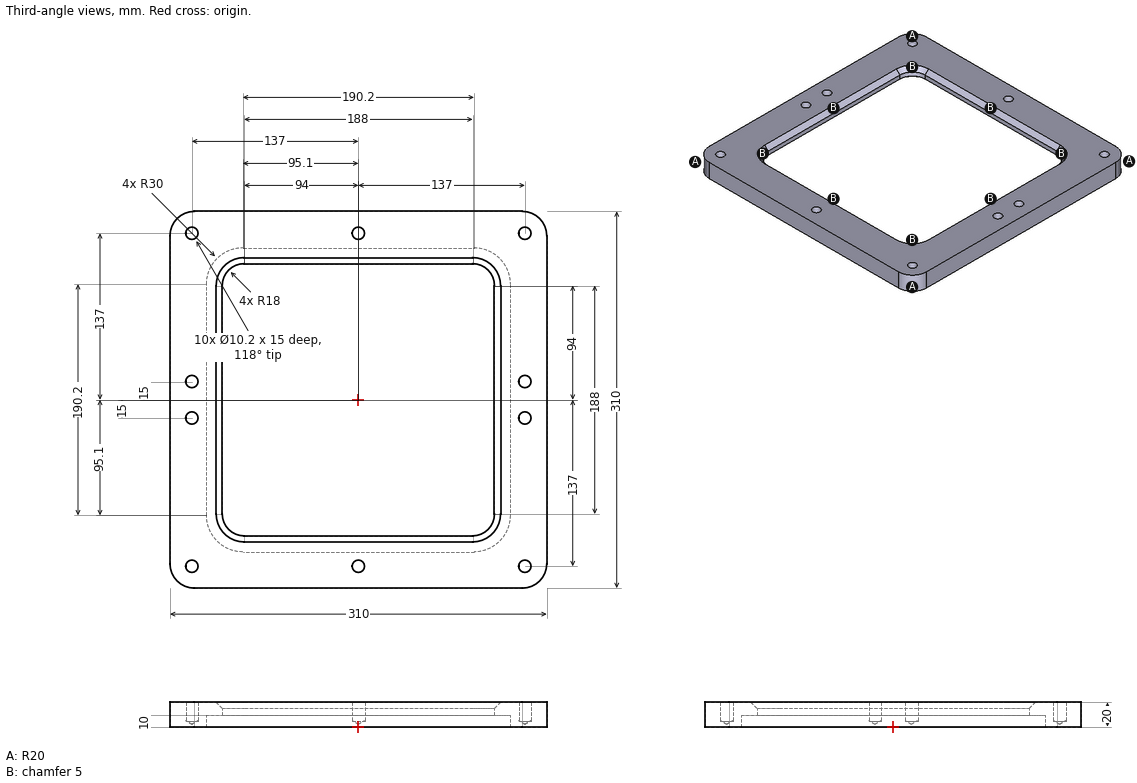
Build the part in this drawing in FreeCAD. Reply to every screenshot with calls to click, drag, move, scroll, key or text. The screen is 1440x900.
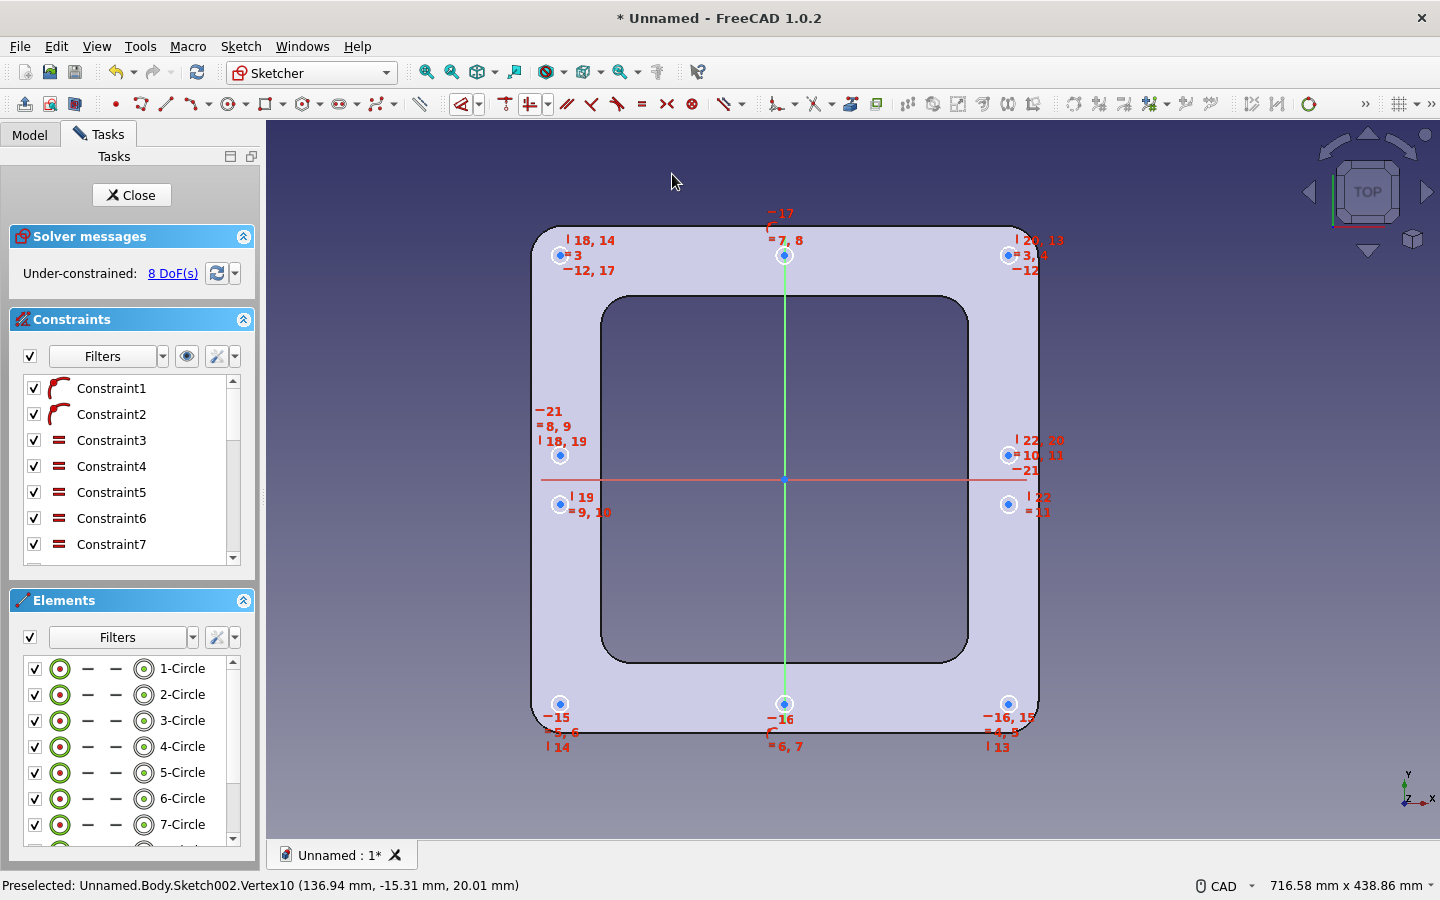
click(560, 505)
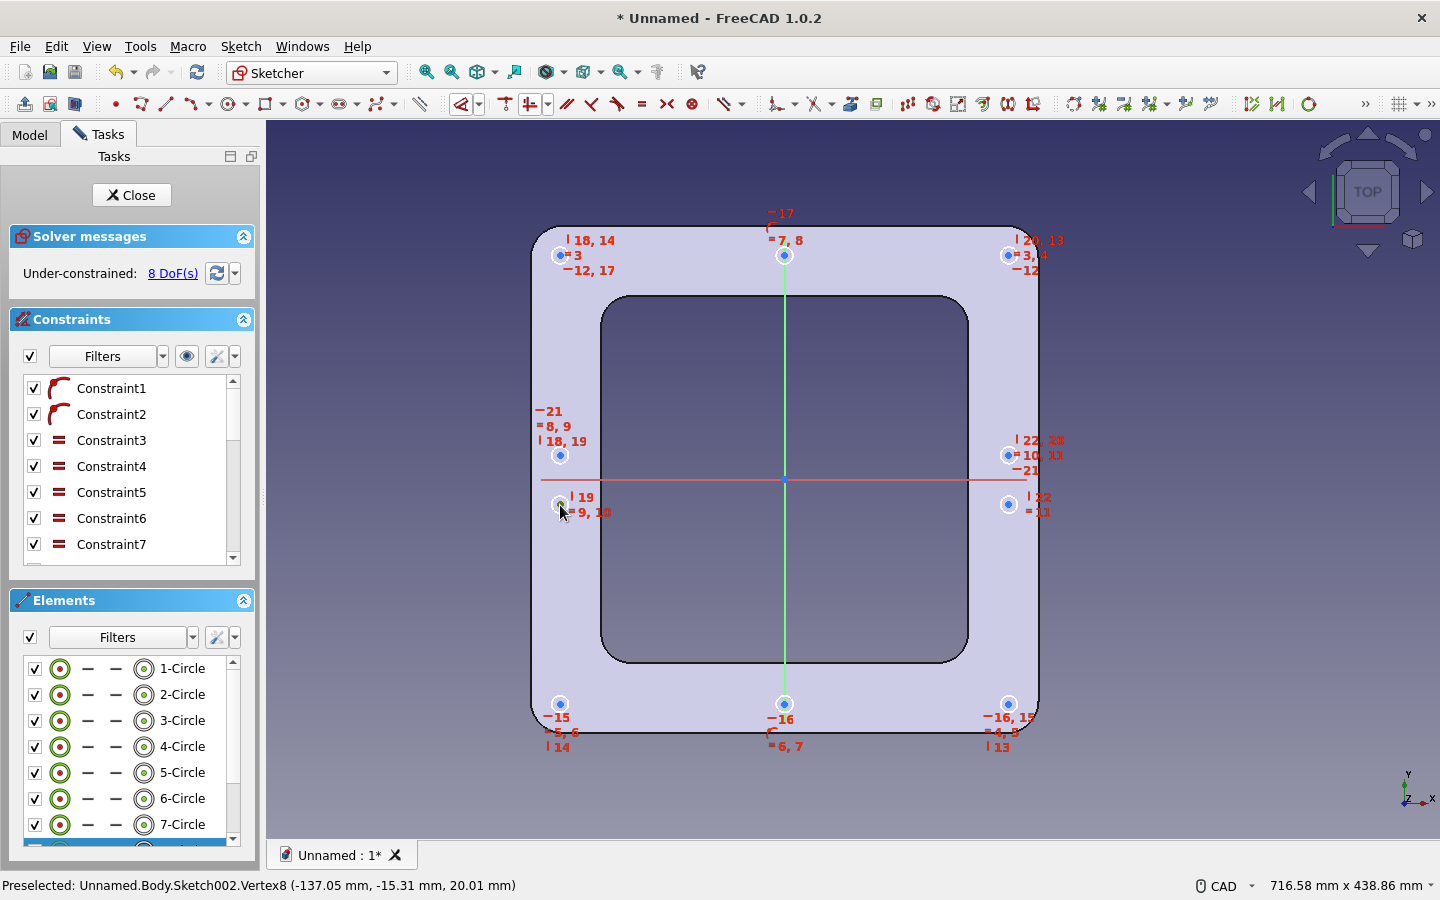
click(1009, 505)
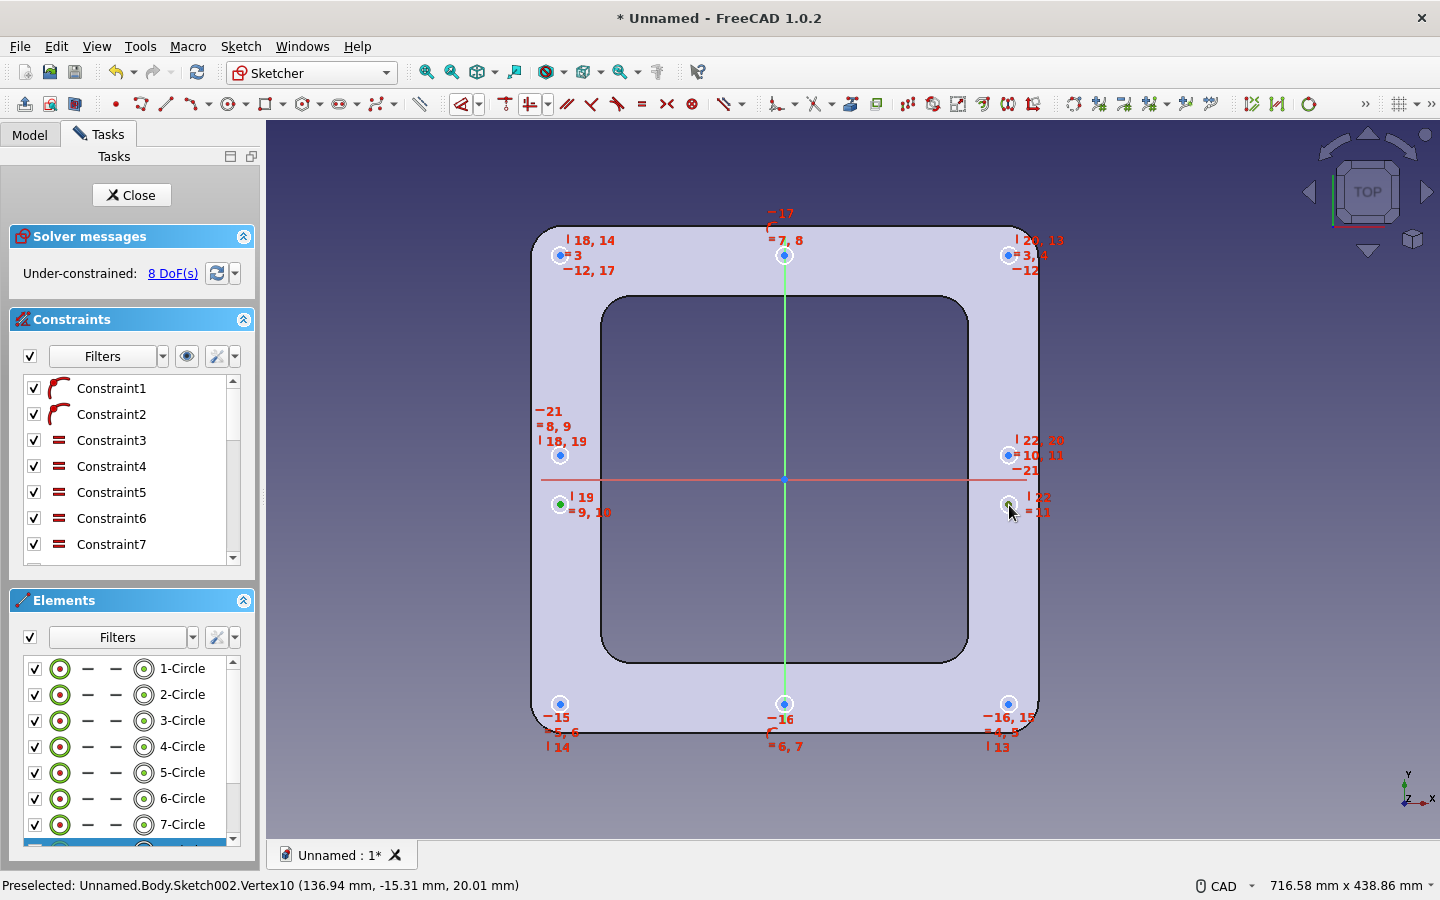
click(548, 104)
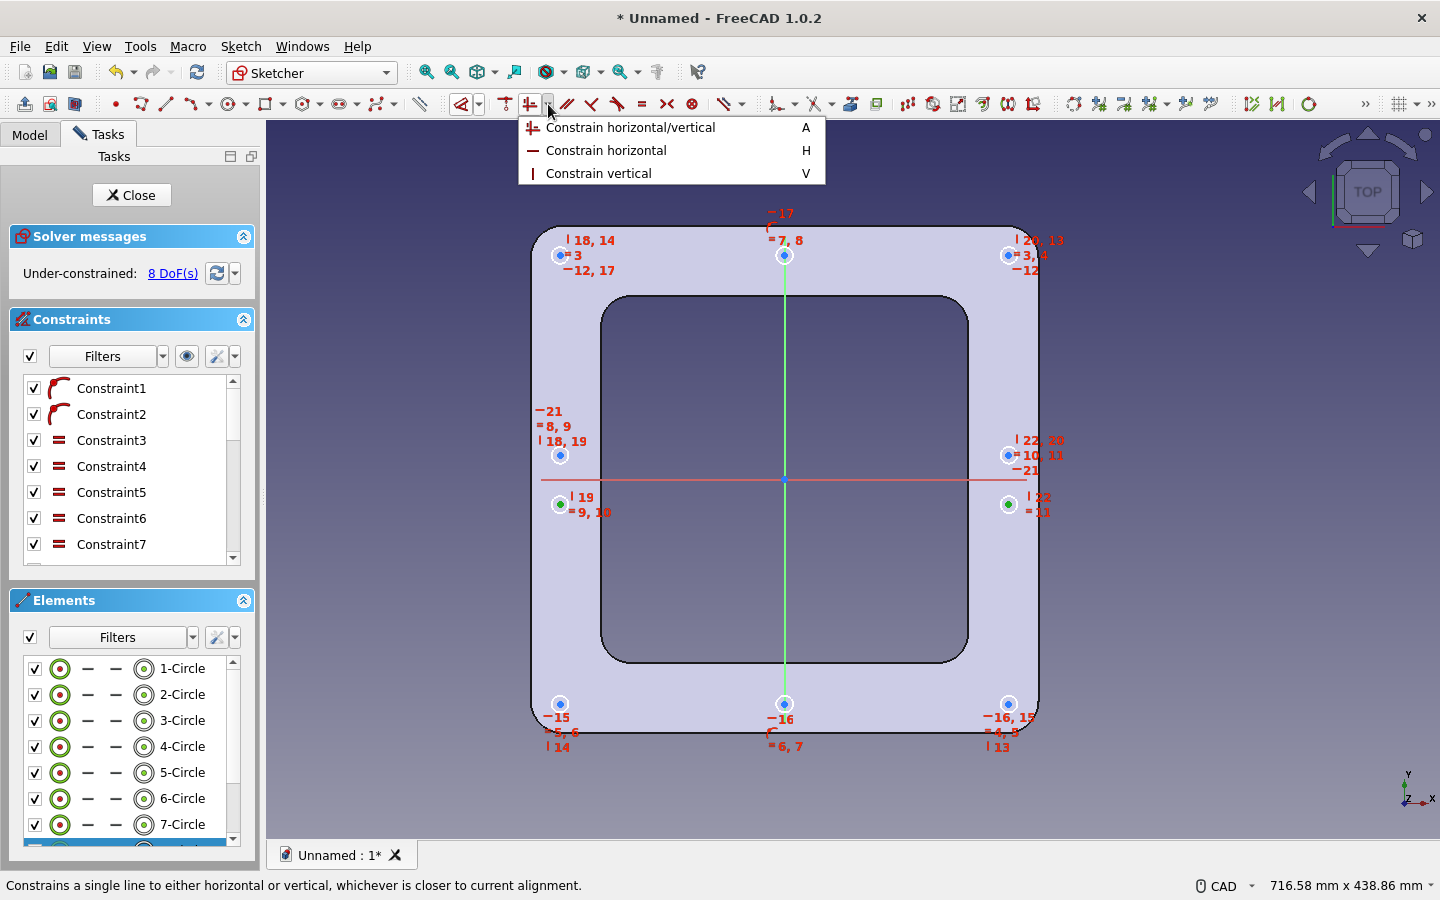
click(672, 150)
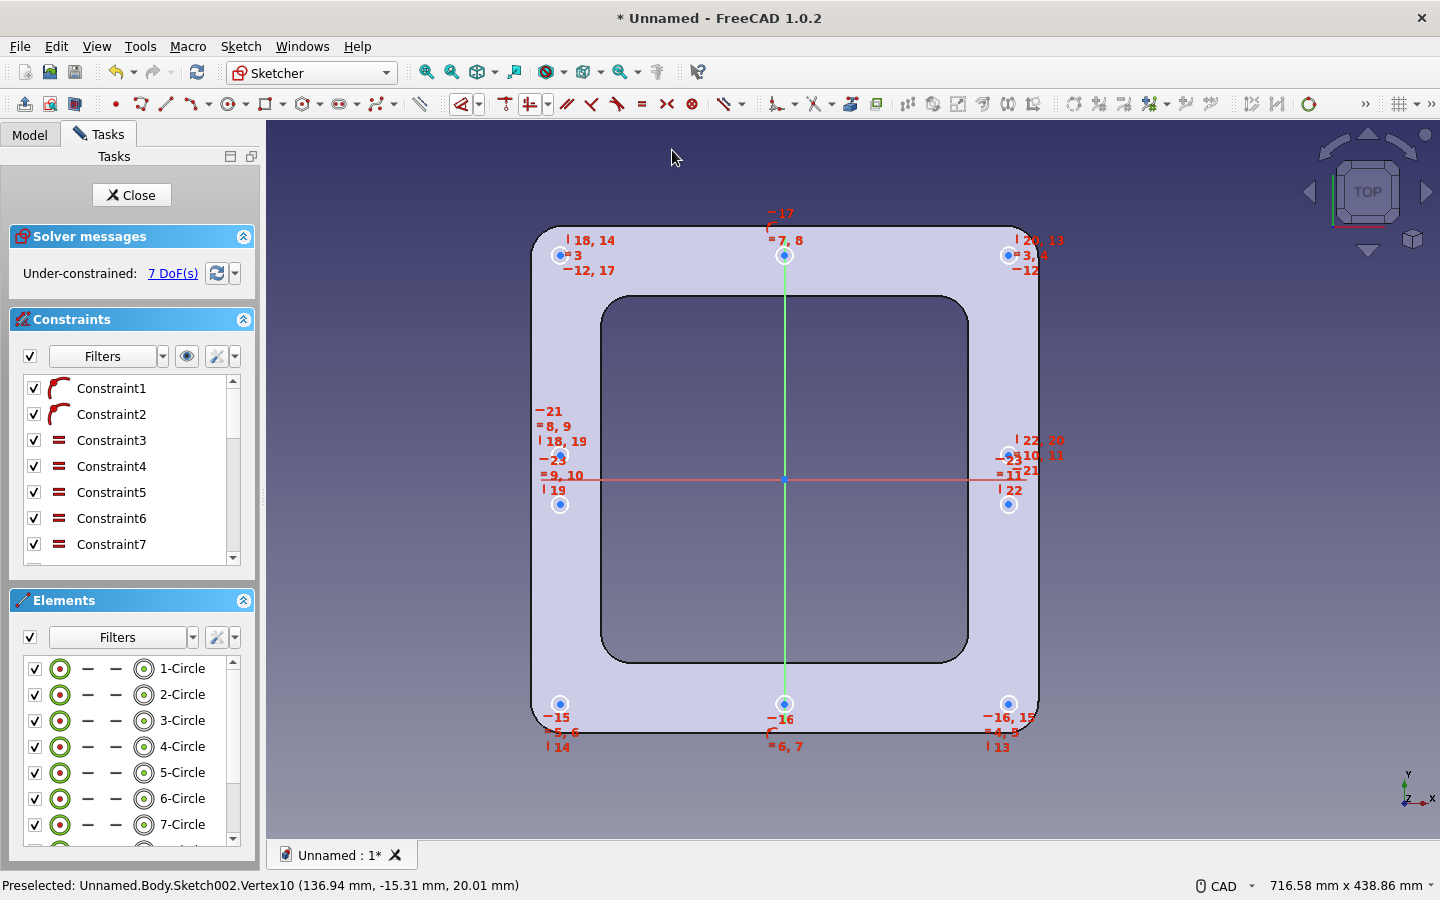
scroll(560, 247, up, 5)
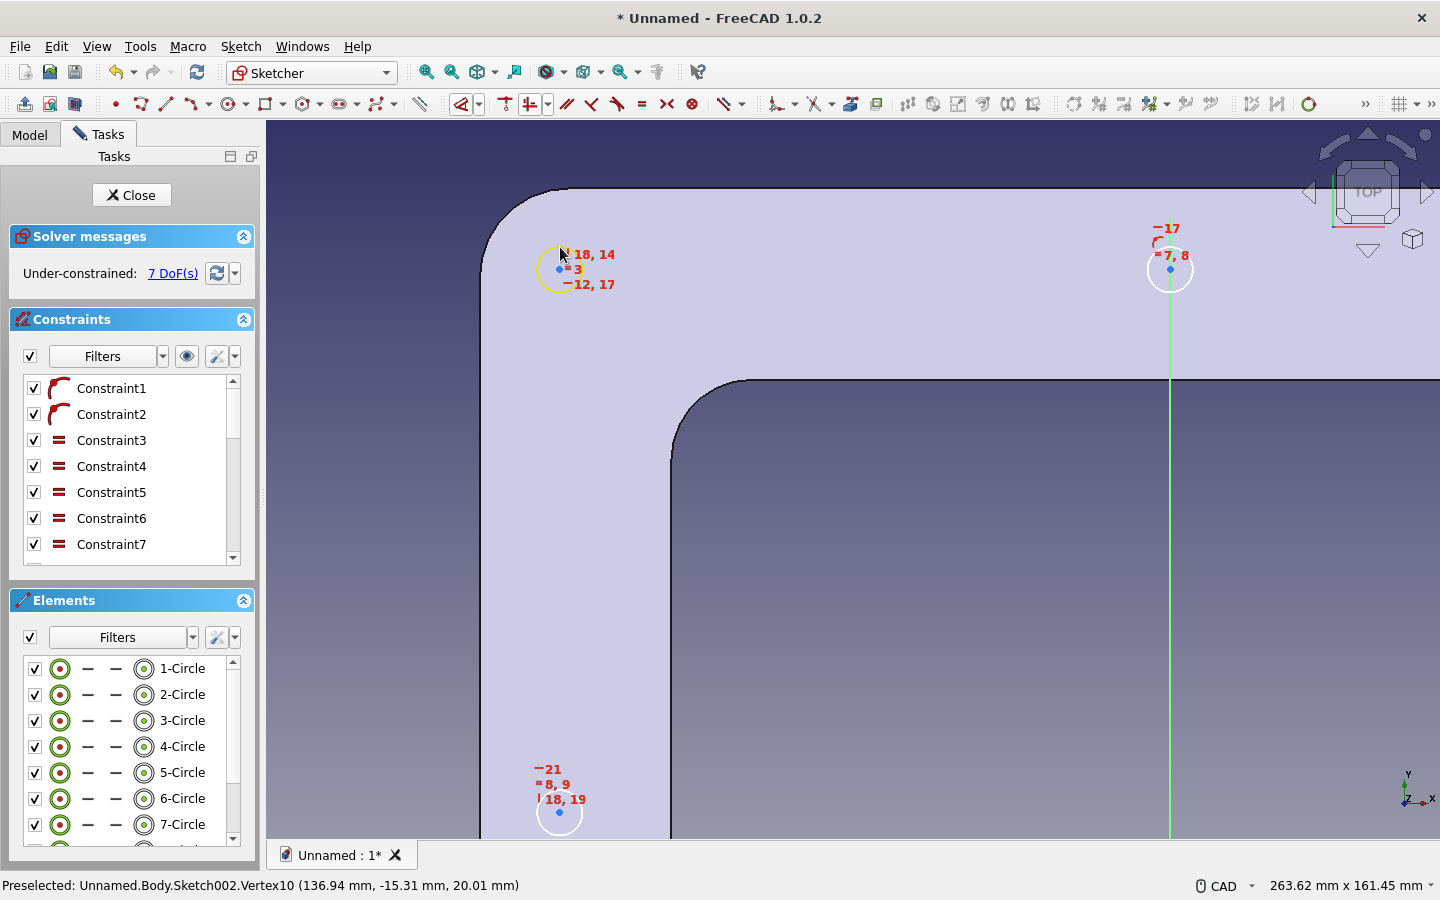
click(560, 247)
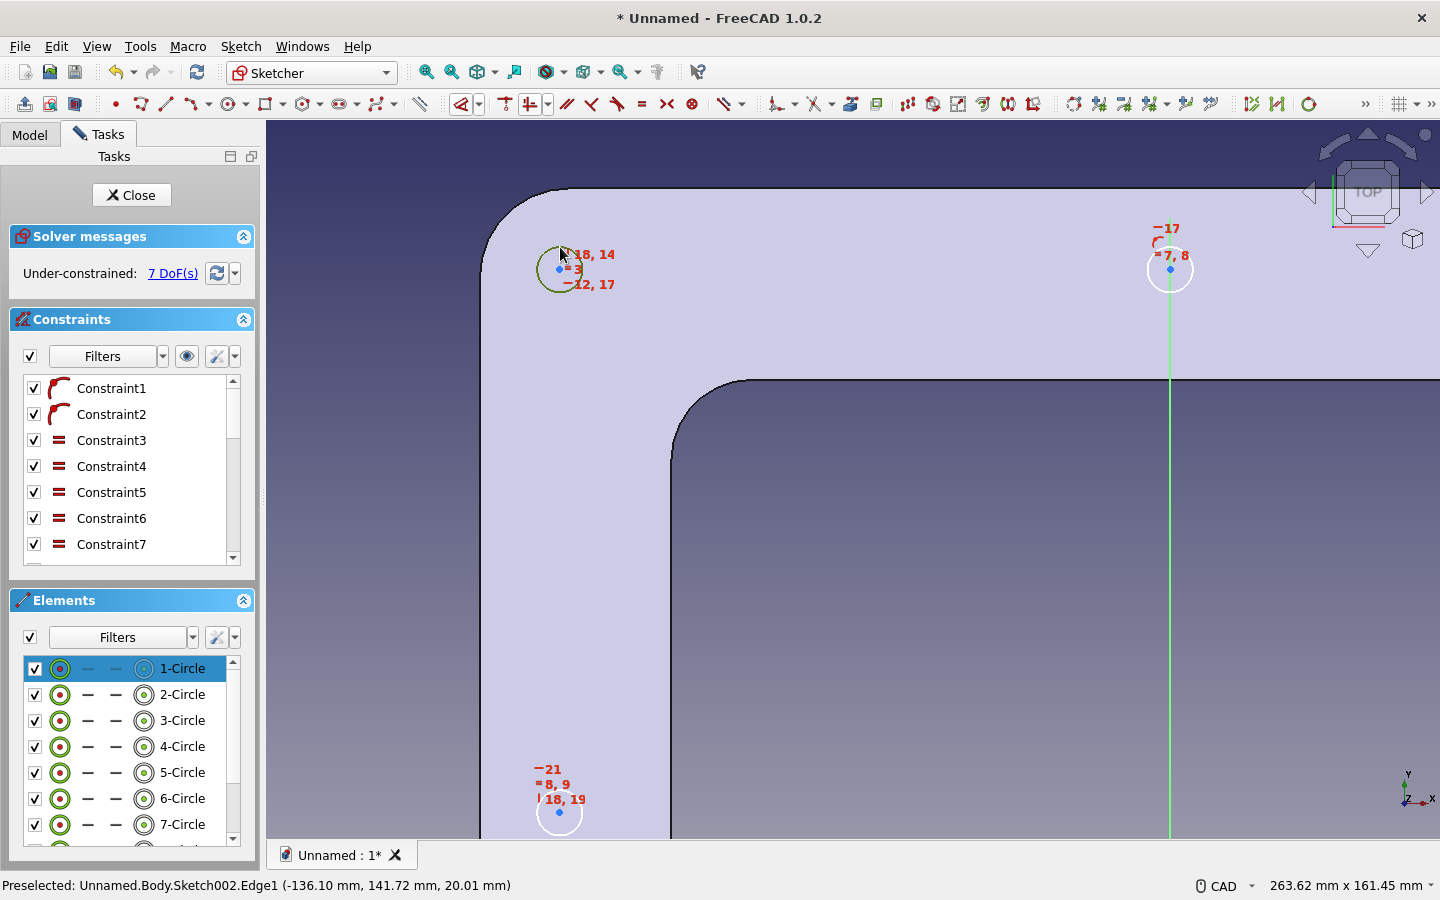
click(478, 104)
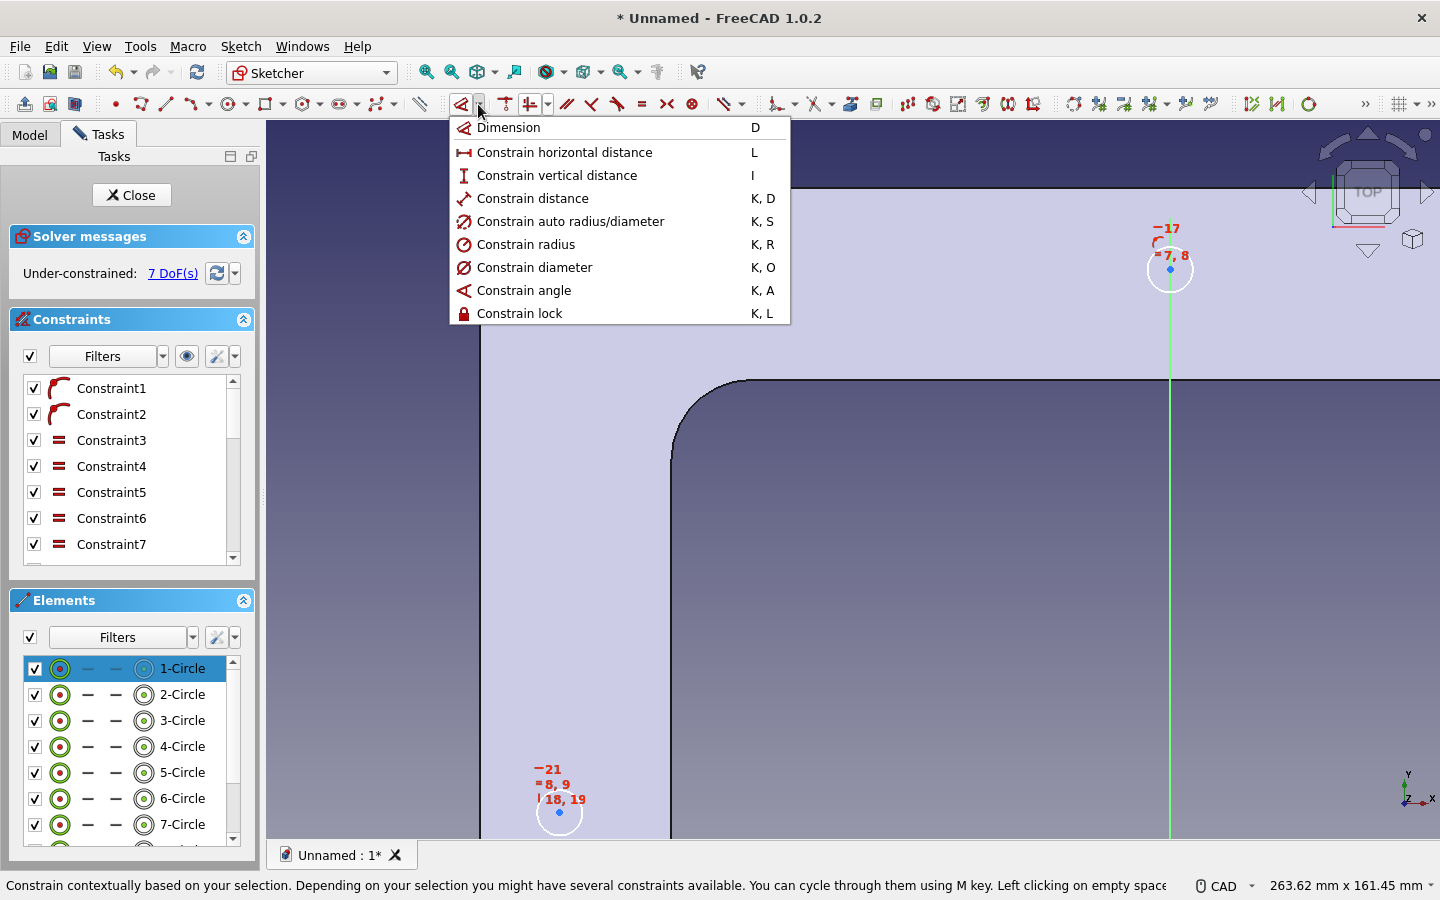
click(620, 268)